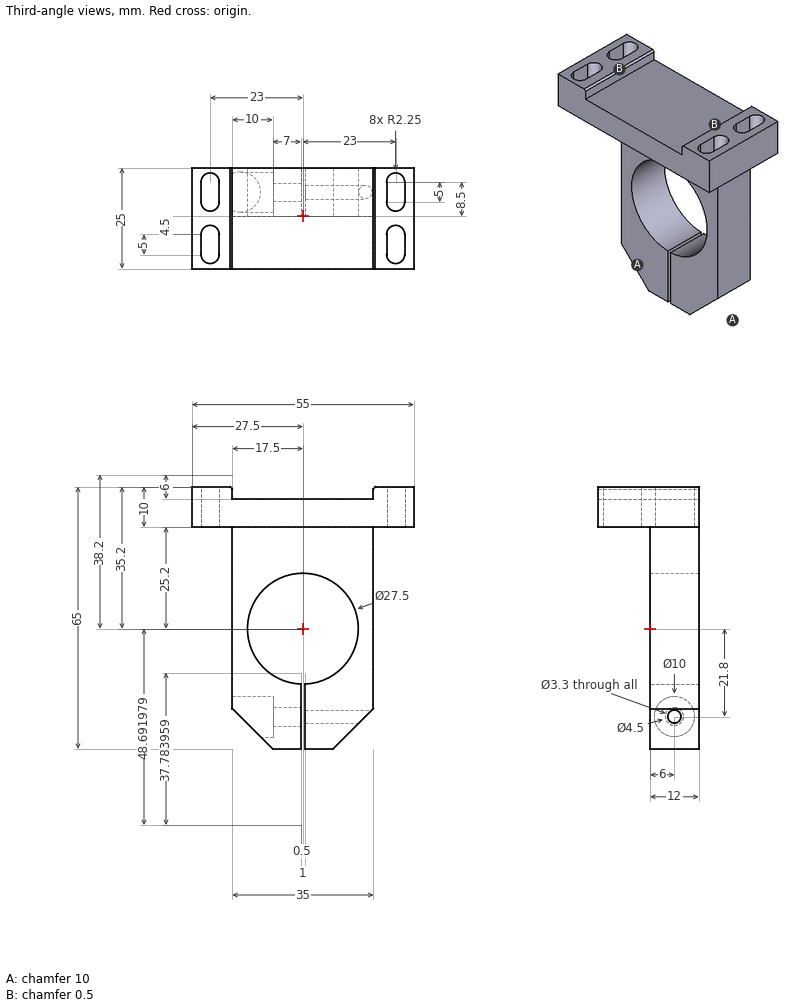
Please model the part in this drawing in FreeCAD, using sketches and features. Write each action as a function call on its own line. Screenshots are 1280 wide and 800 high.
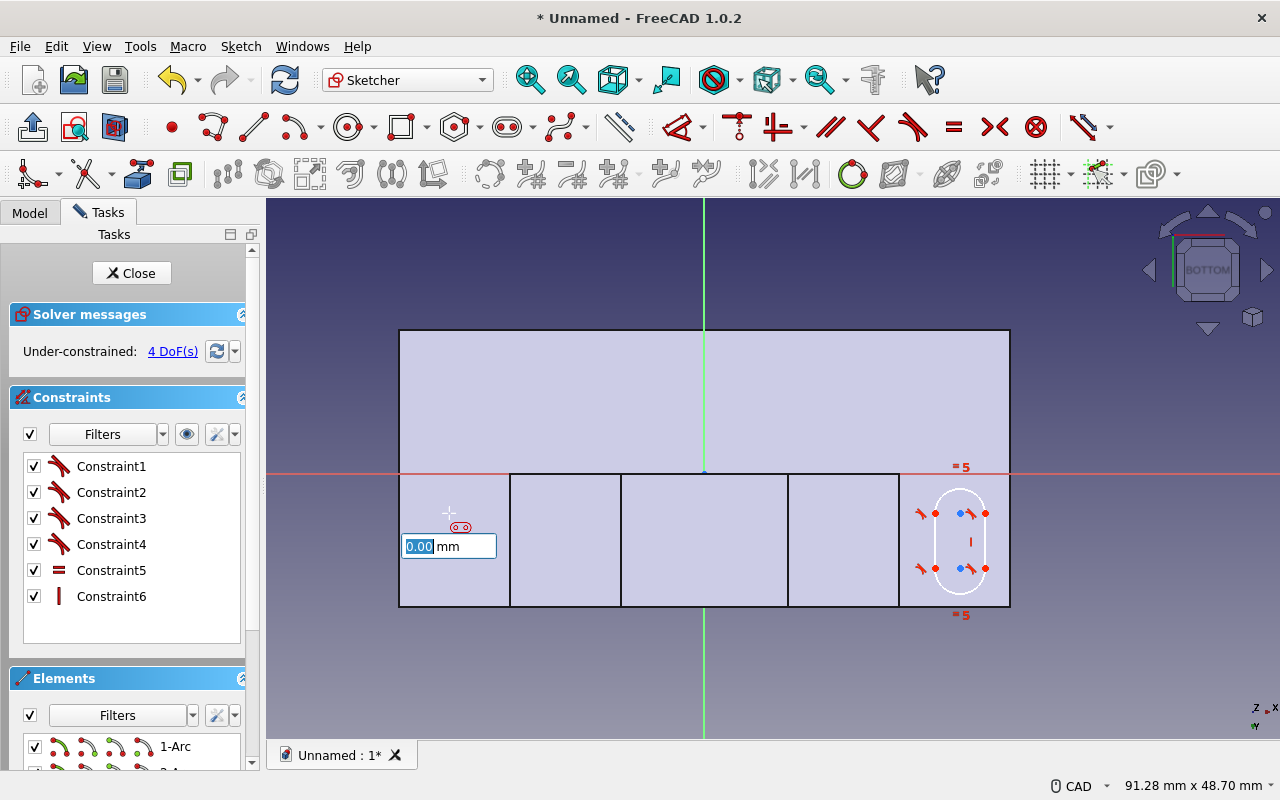
click(474, 541)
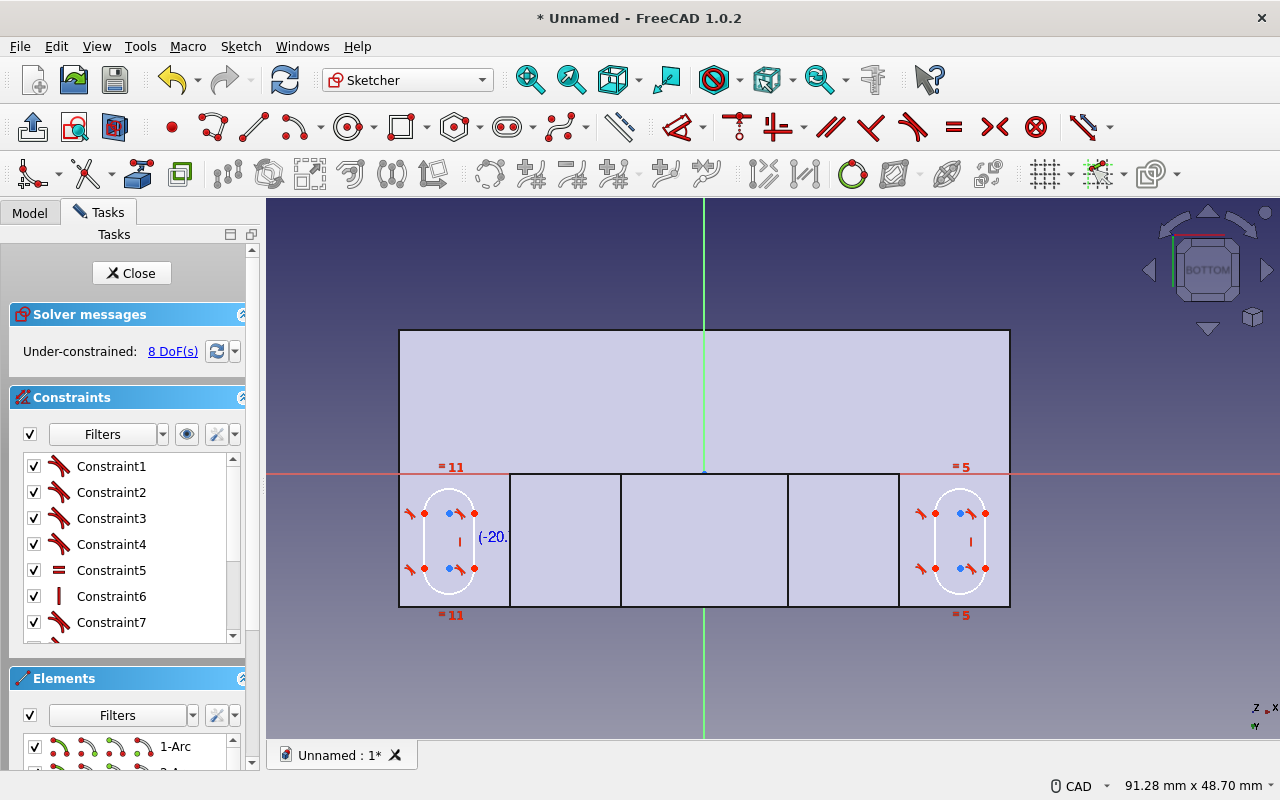
click(449, 424)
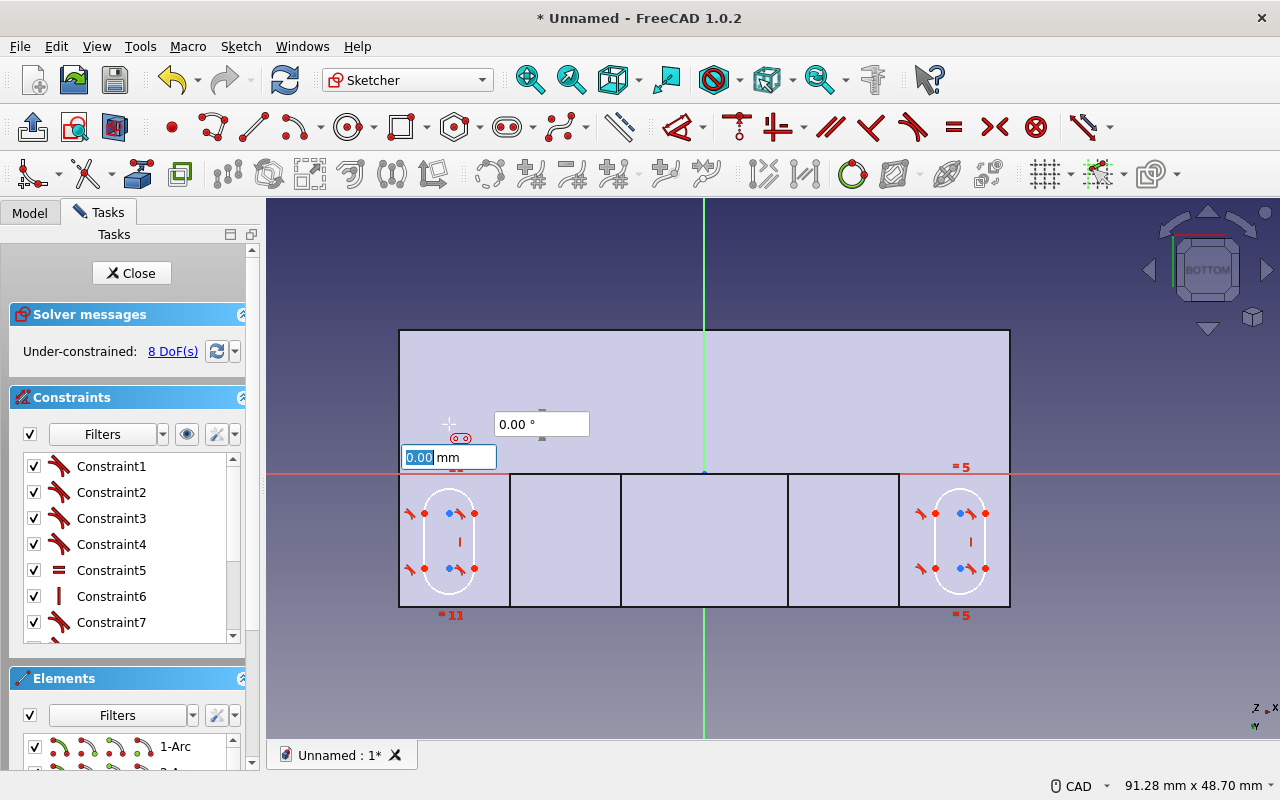
click(449, 369)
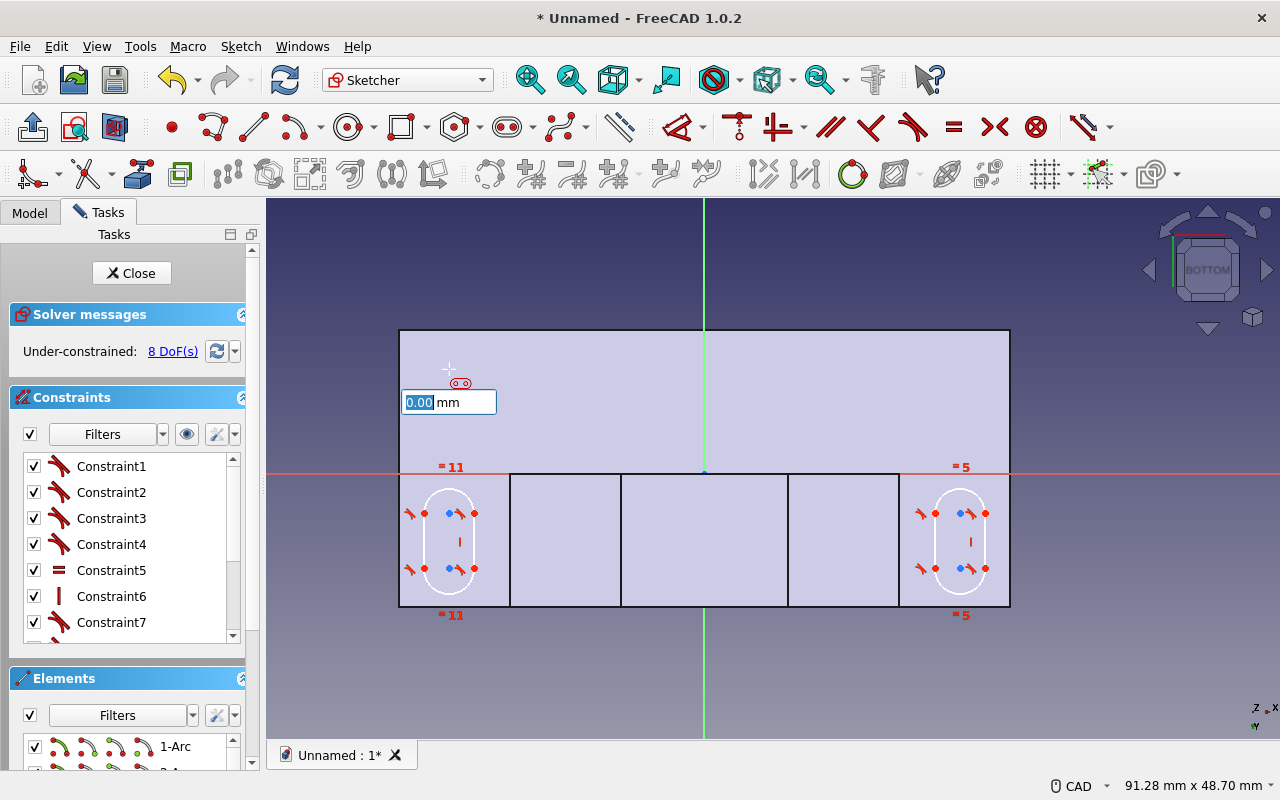
click(474, 396)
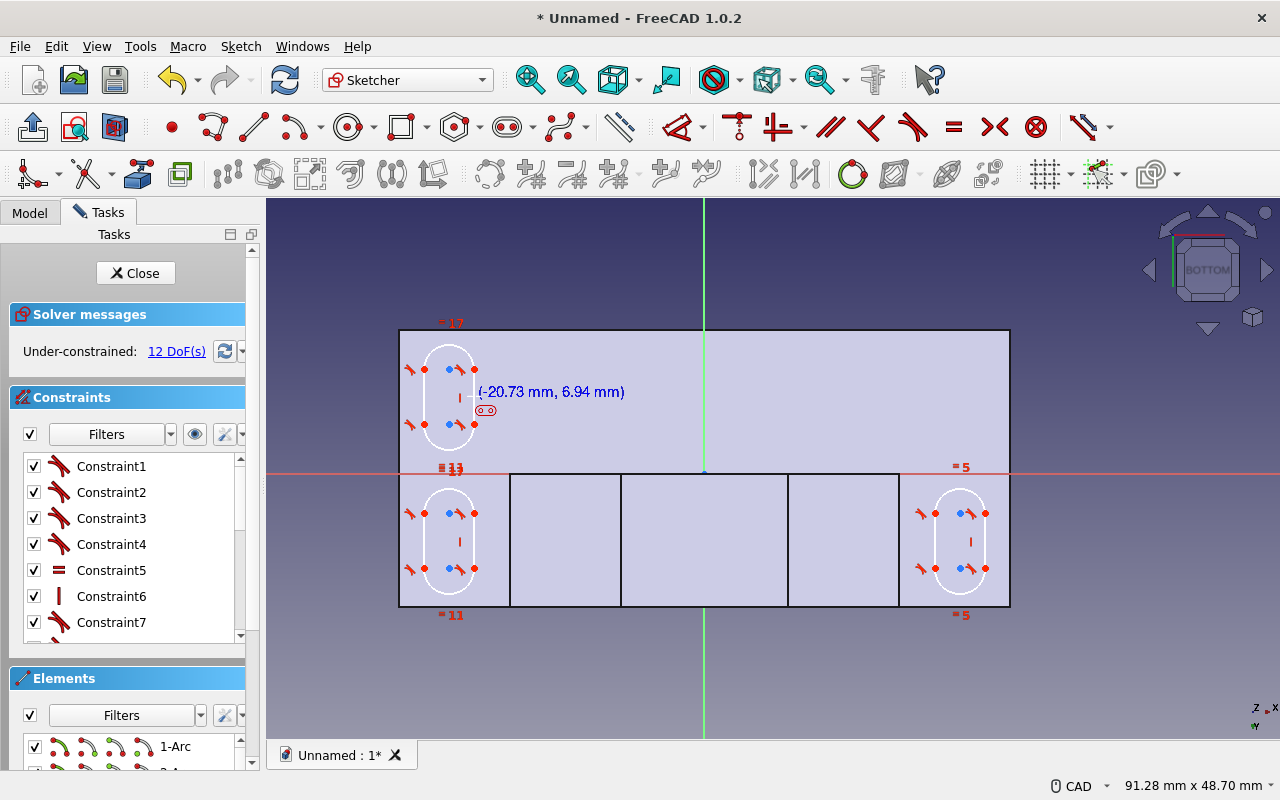
click(960, 424)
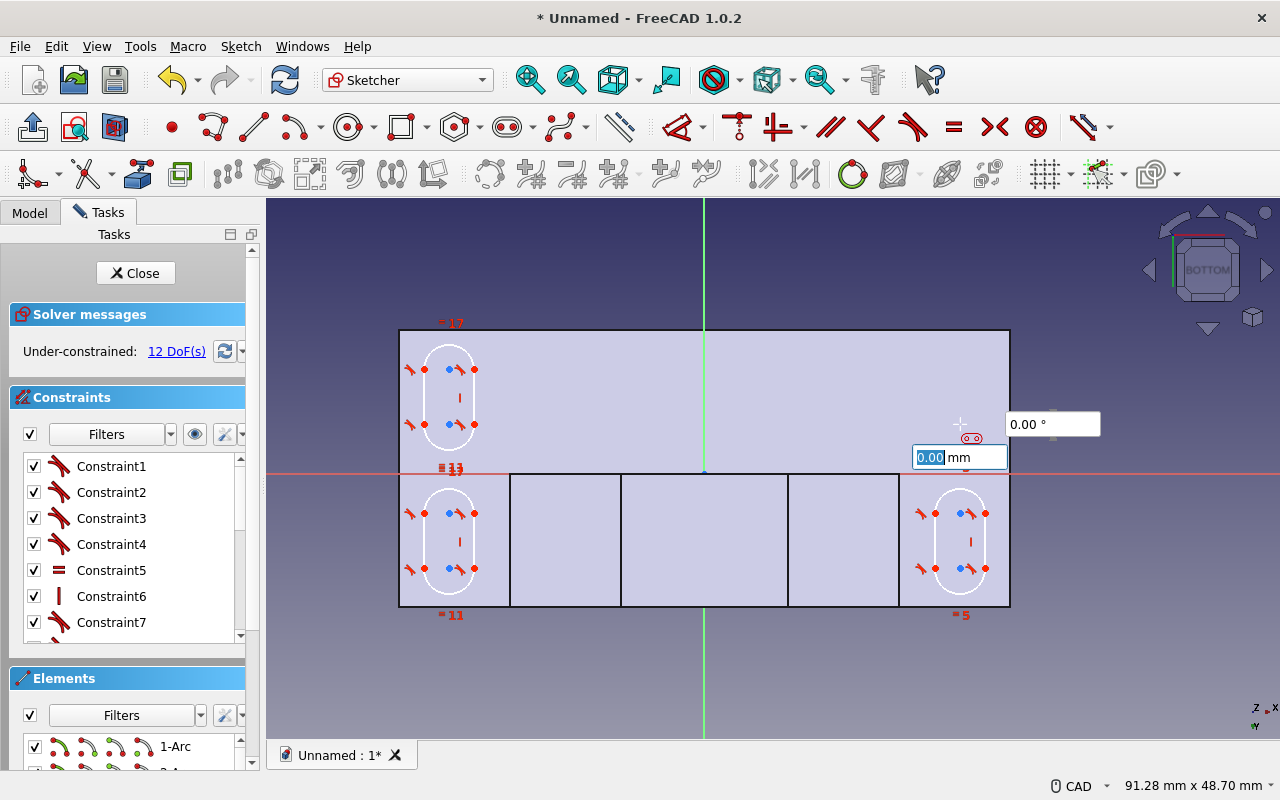
click(960, 369)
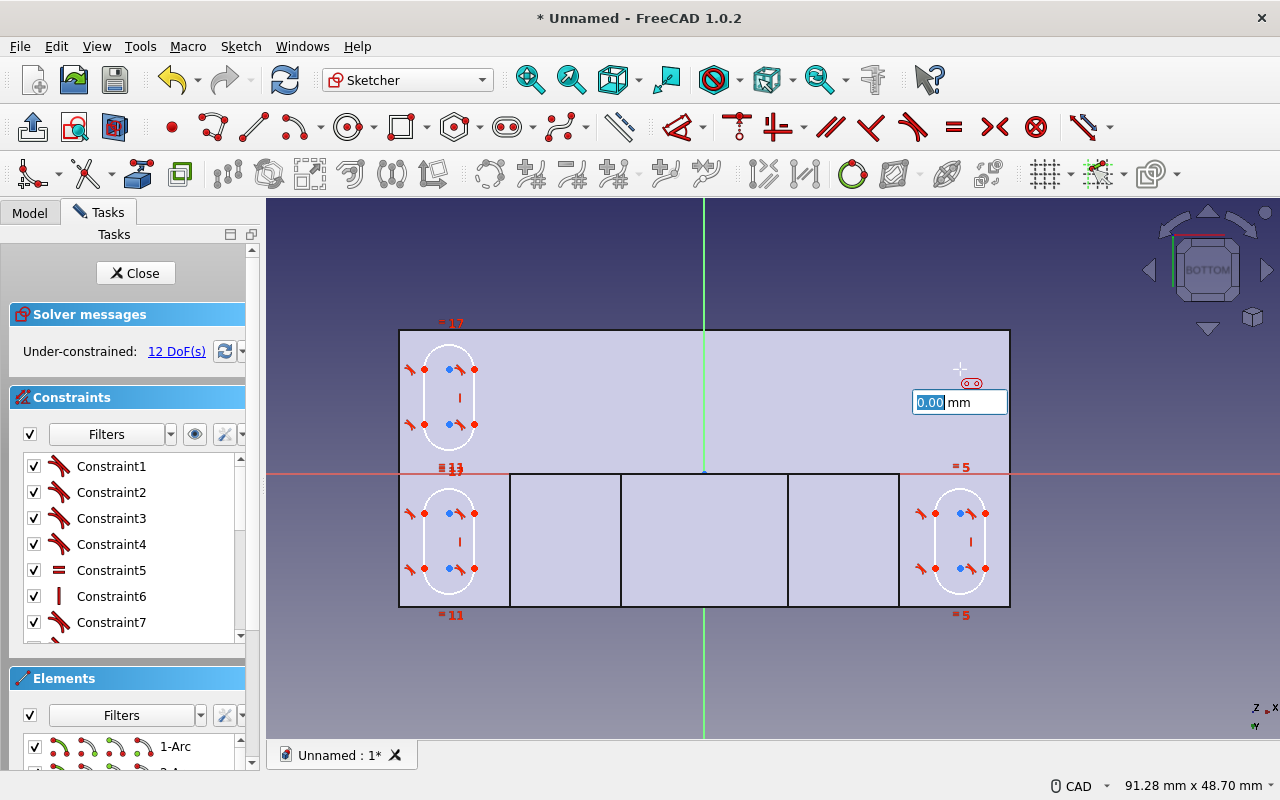
click(935, 396)
key(Escape)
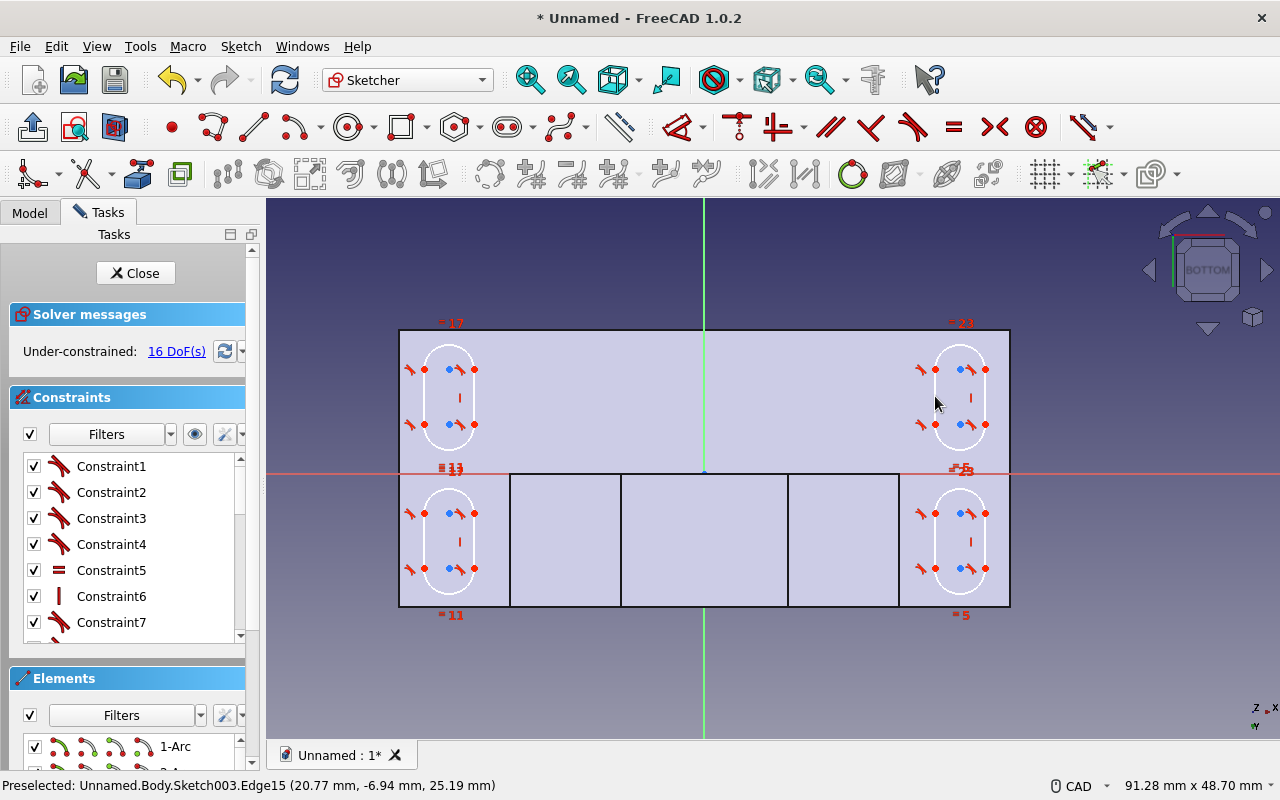
click(945, 589)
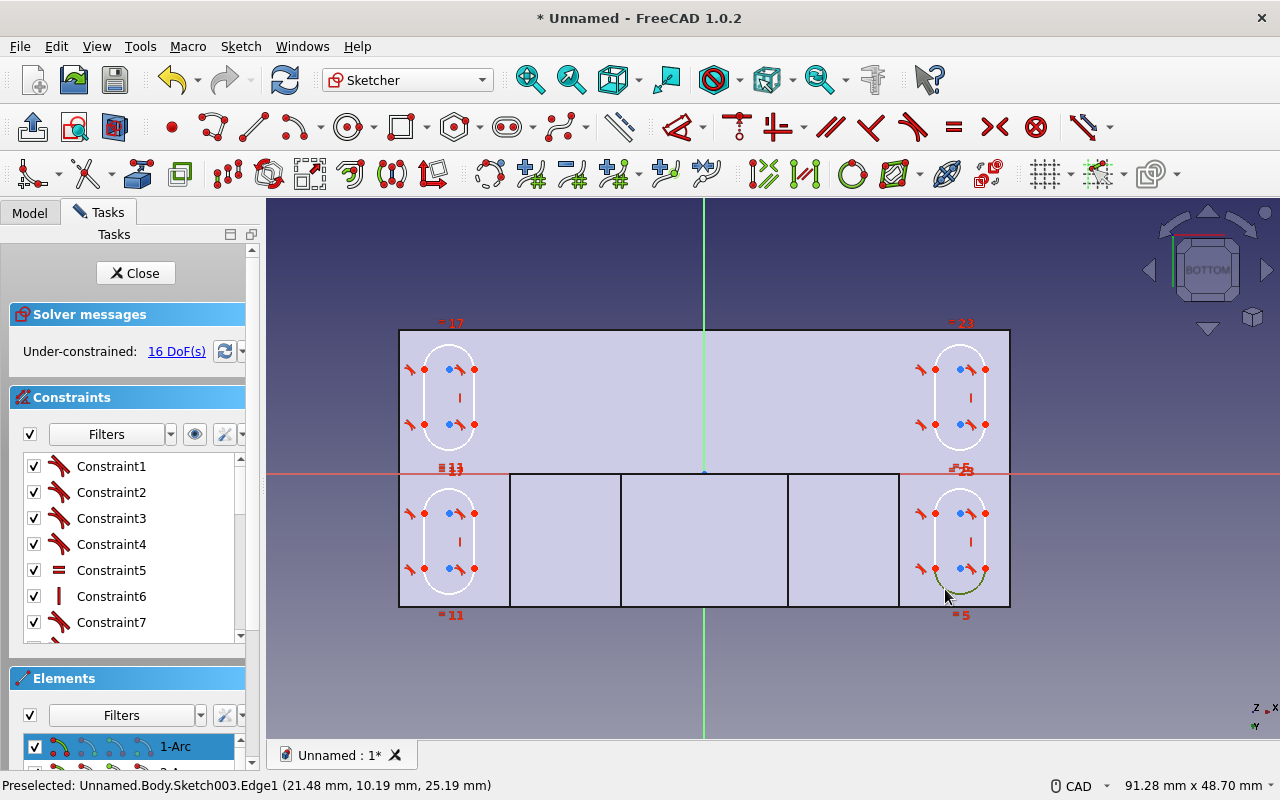
click(434, 589)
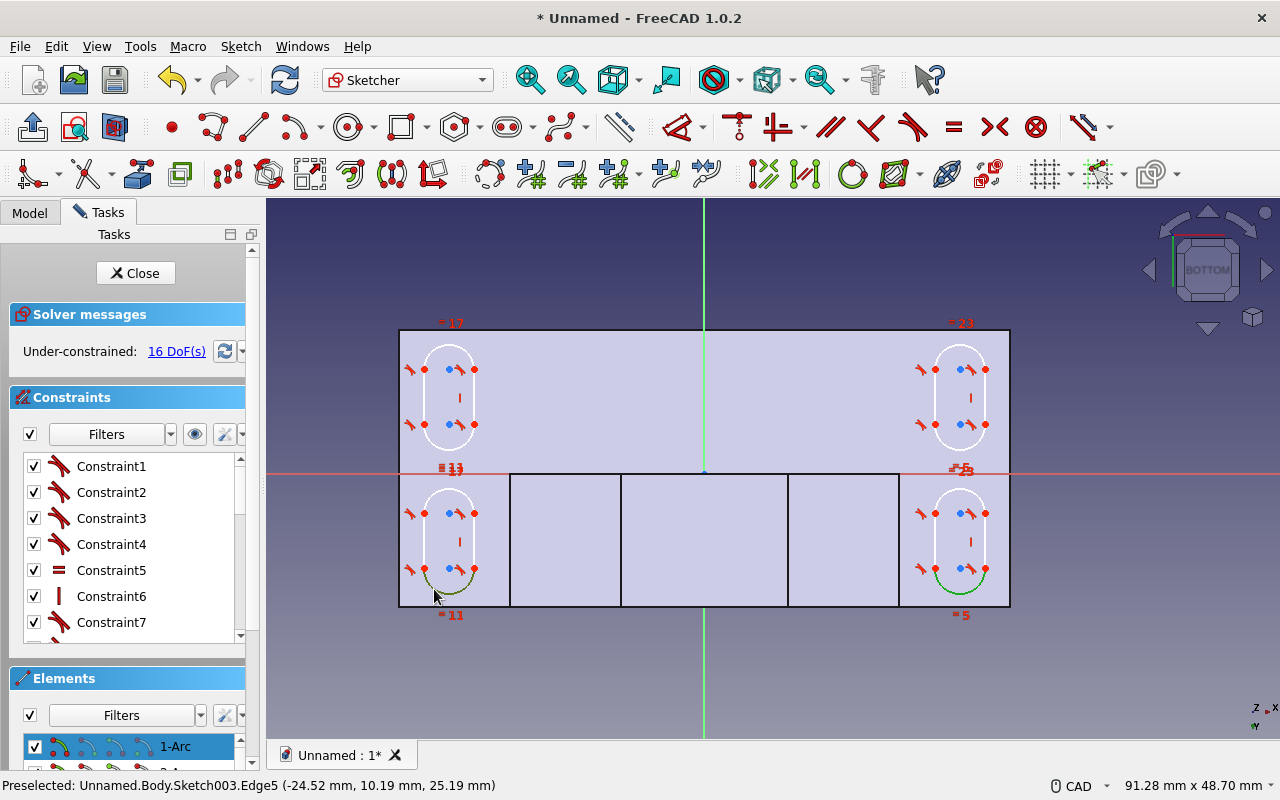
click(434, 445)